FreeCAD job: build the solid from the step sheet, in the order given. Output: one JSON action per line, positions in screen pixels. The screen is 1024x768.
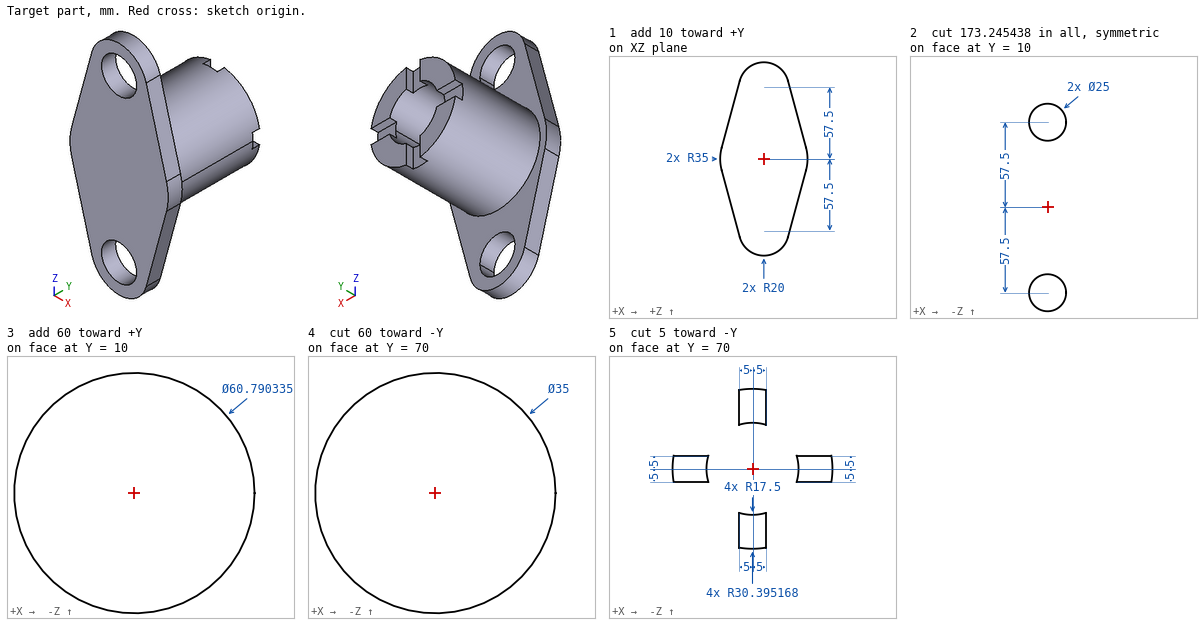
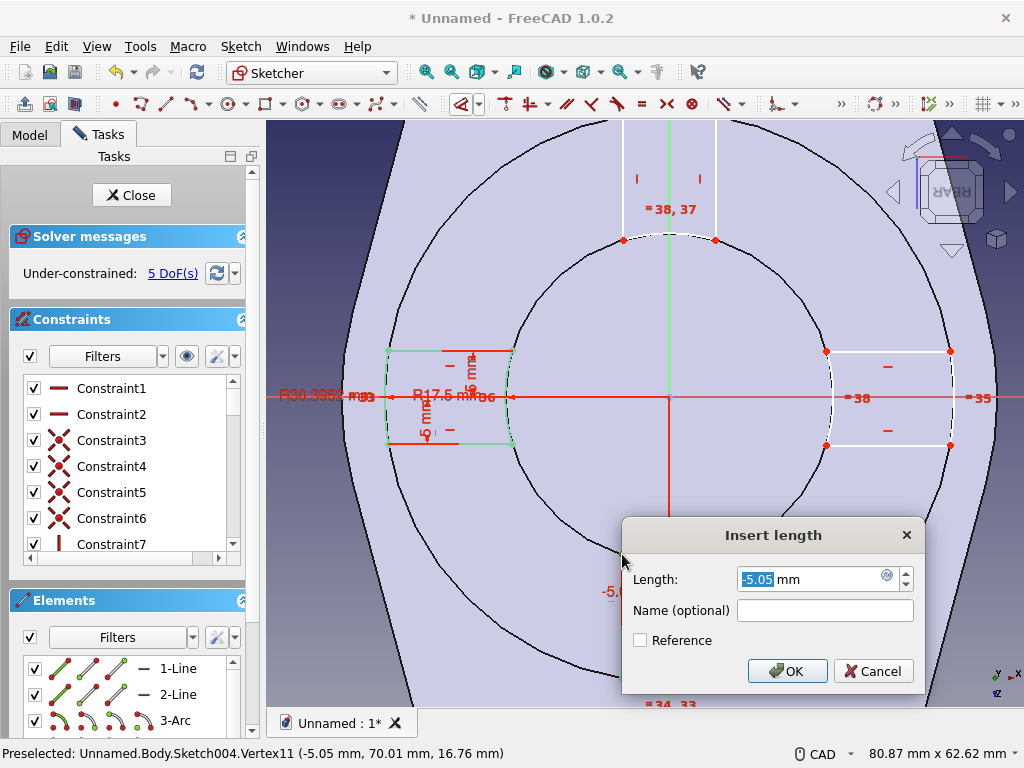
{"action": "type", "text": "-5"}
{"action": "key", "text": "Return"}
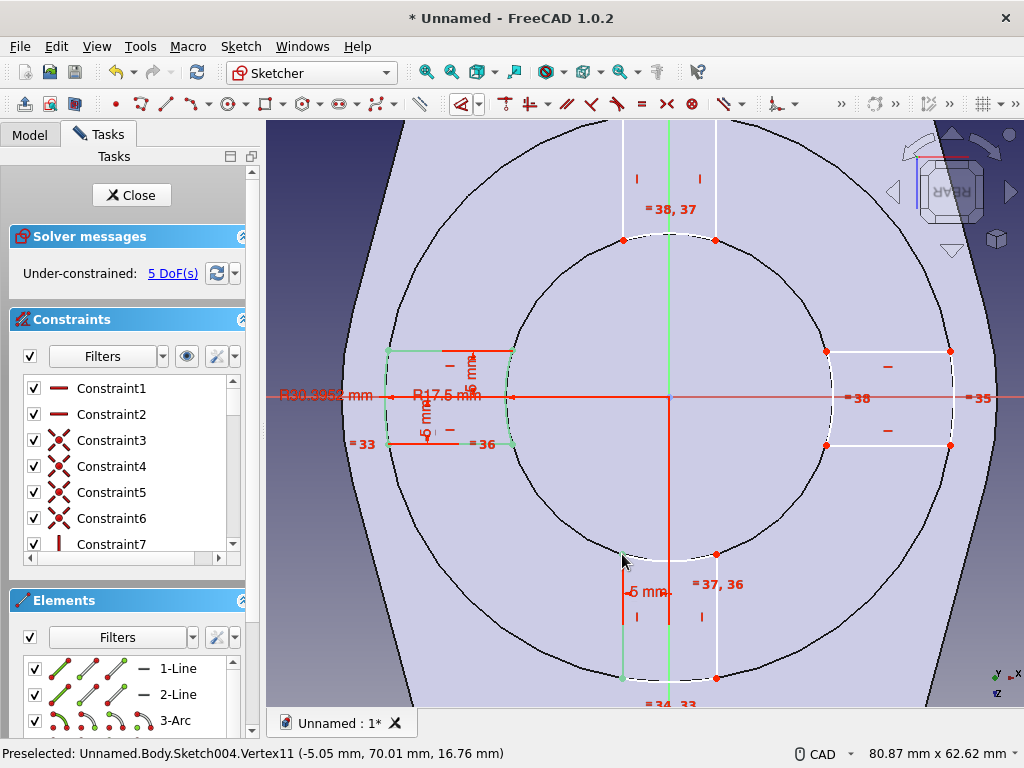
{"action": "left_click", "coordinate": [717, 678]}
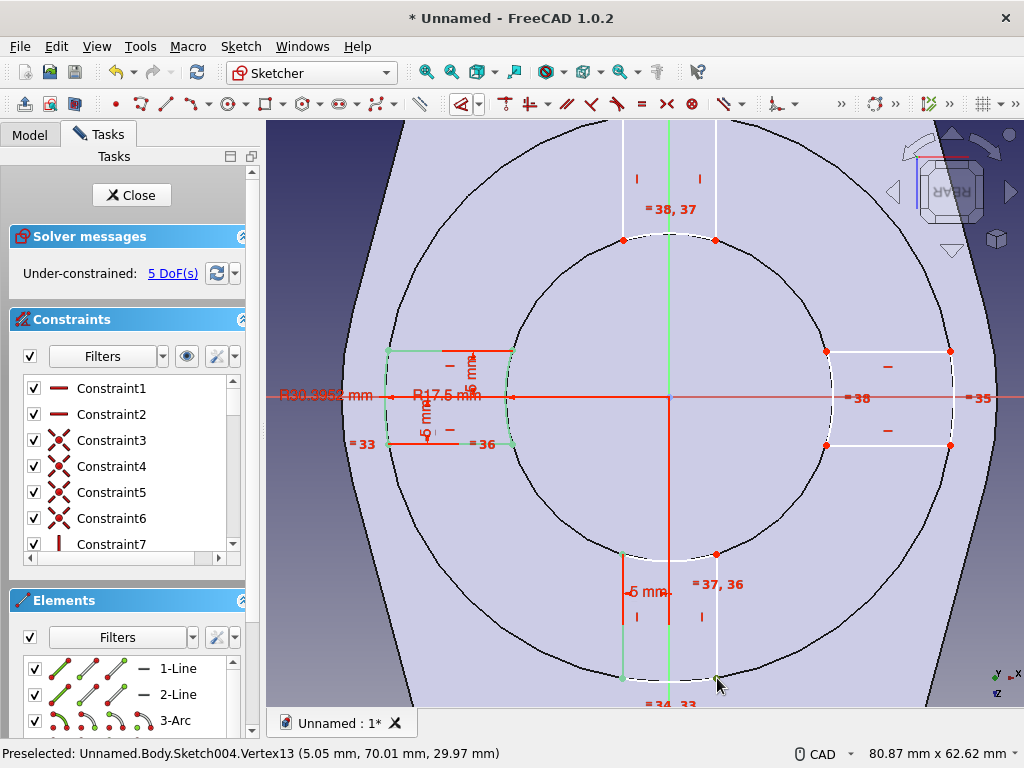
{"action": "left_click", "coordinate": [478, 104]}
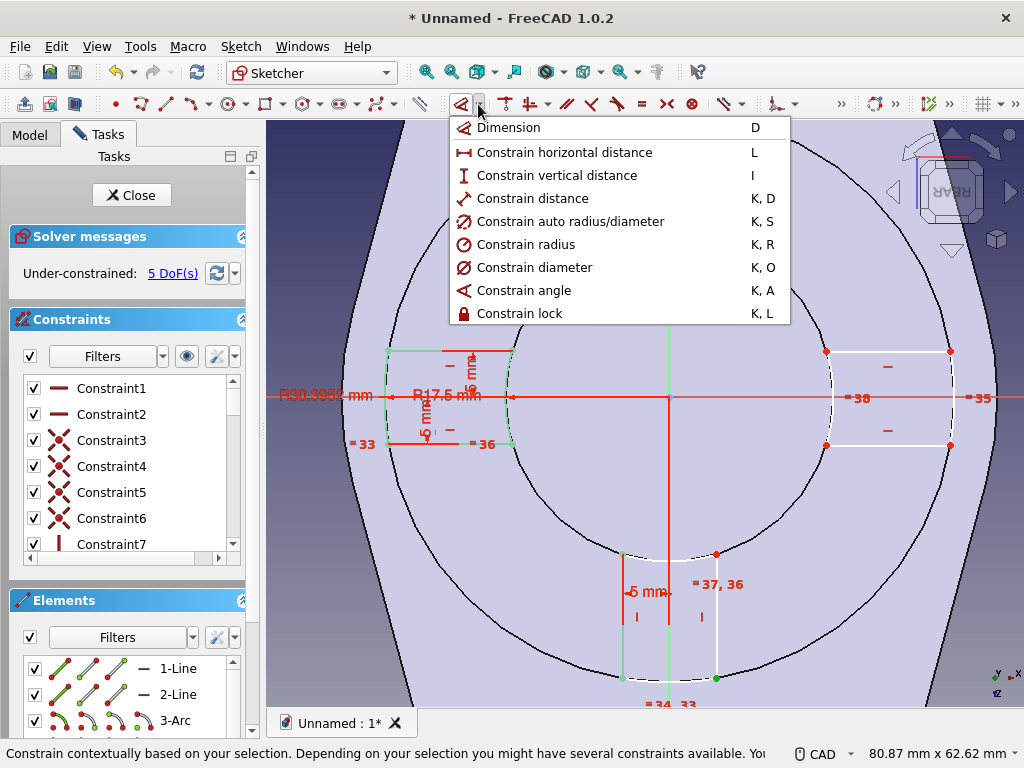
{"action": "left_click", "coordinate": [620, 152]}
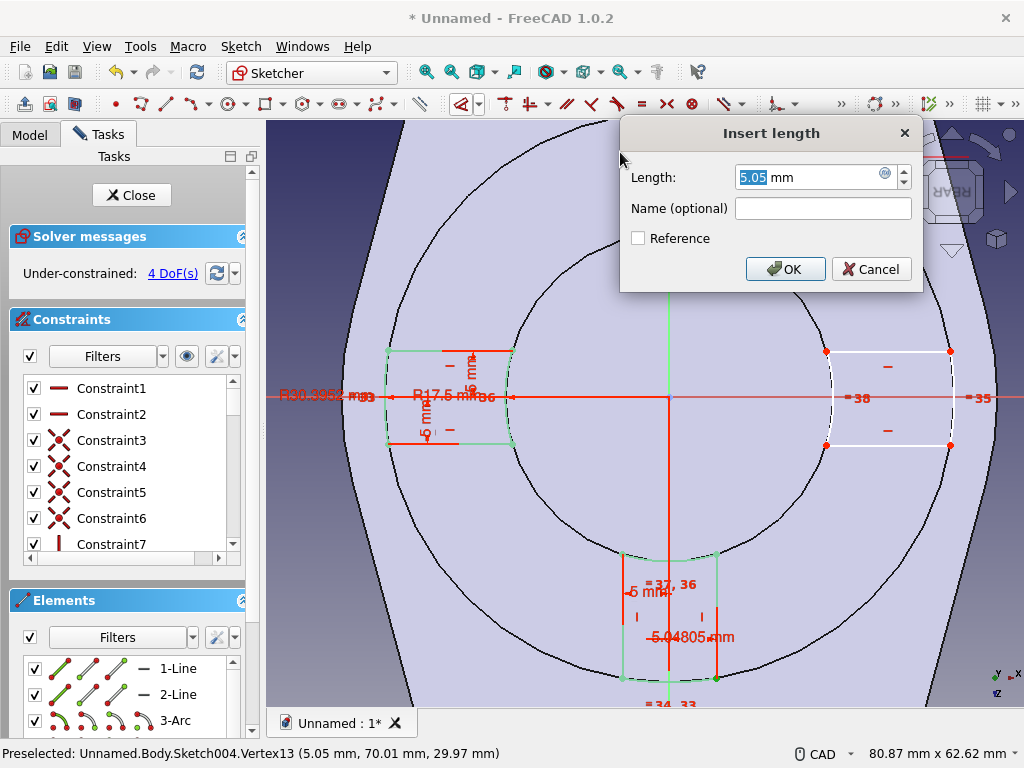
{"action": "type", "text": "5"}
{"action": "key", "text": "Return"}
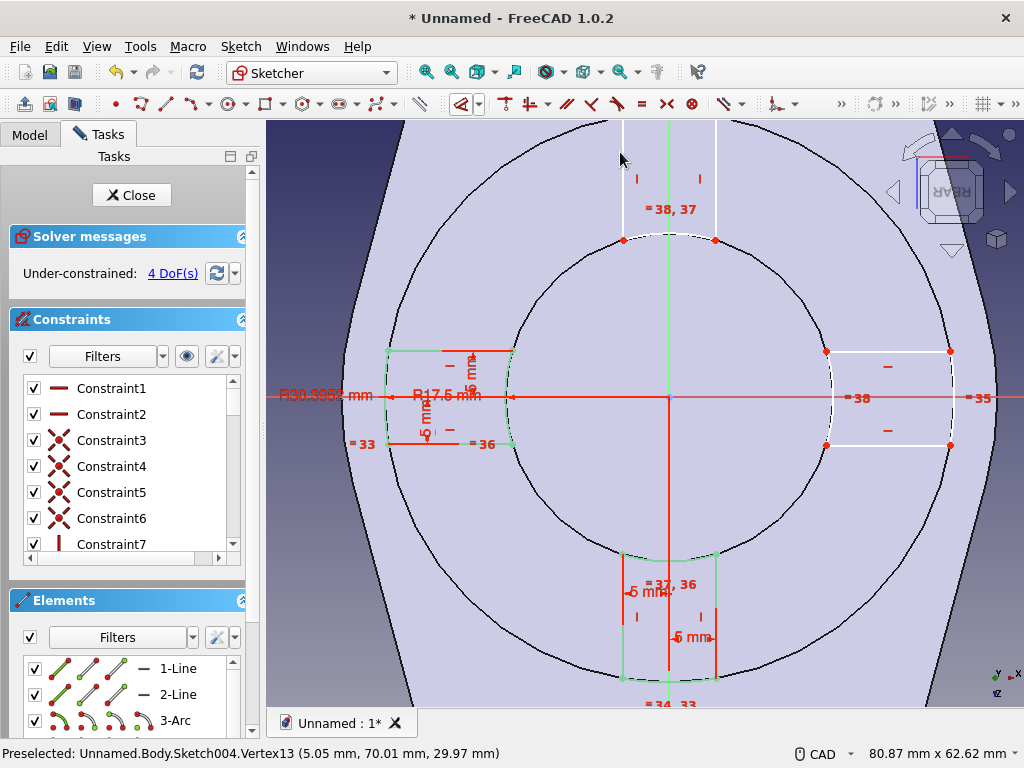
{"action": "scroll", "coordinate": [388, 446], "scroll_direction": "down", "scroll_amount": 2}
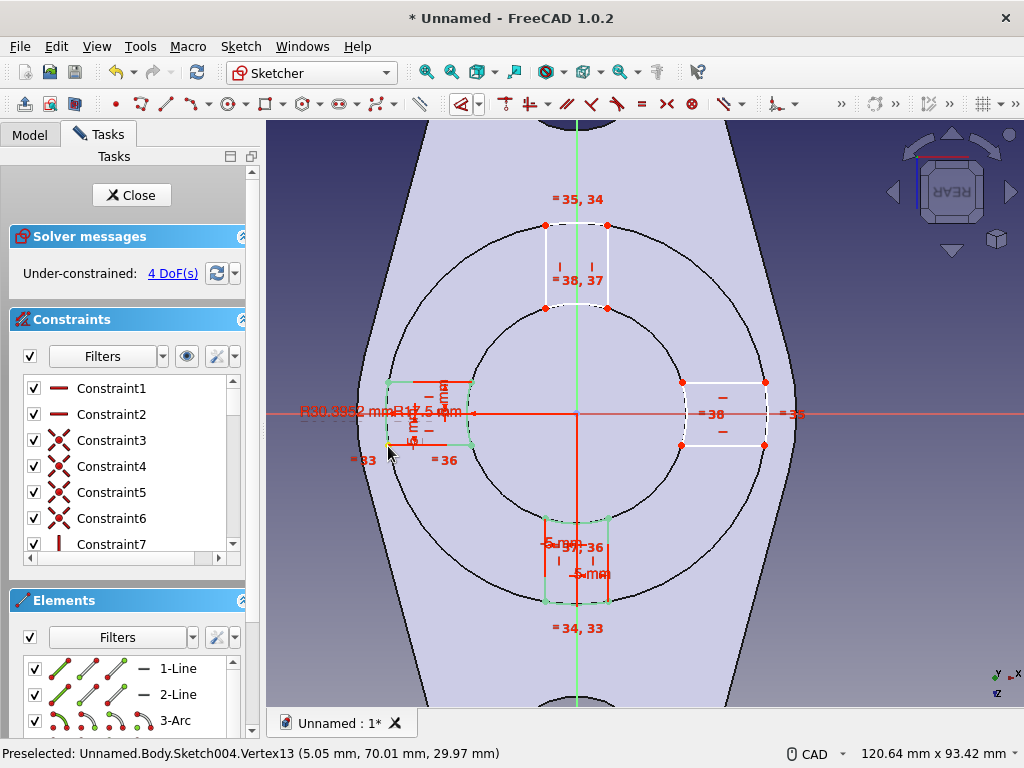
{"action": "scroll", "coordinate": [546, 225], "scroll_direction": "up", "scroll_amount": 2}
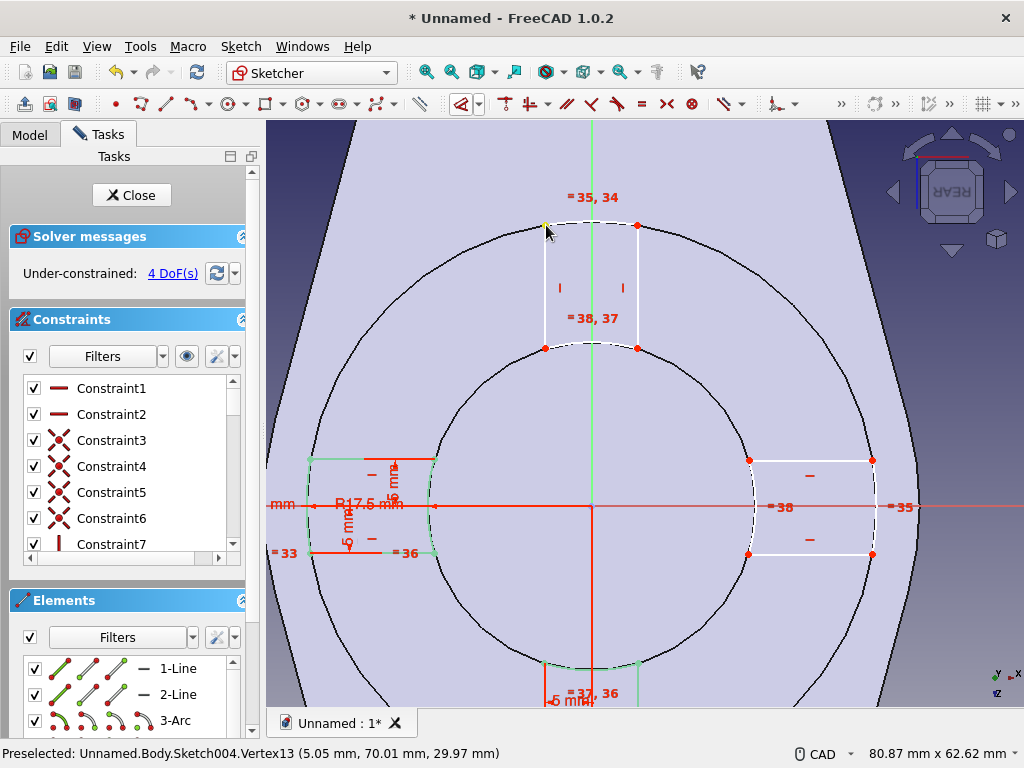
{"action": "left_click", "coordinate": [545, 225]}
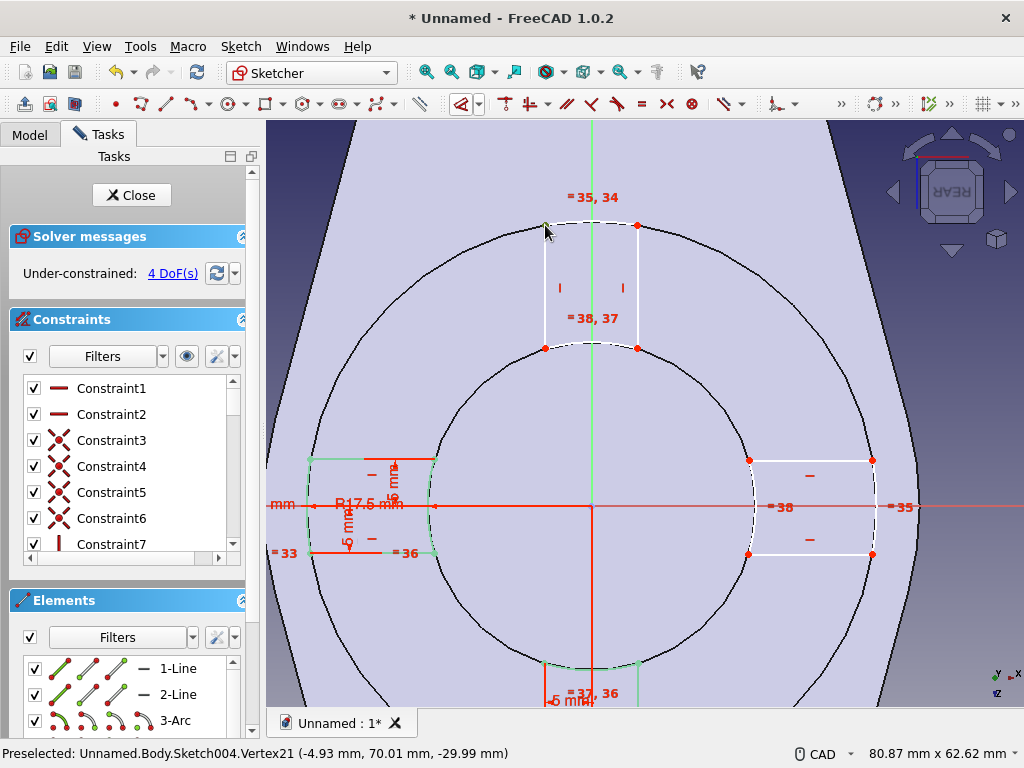
{"action": "key", "text": "l"}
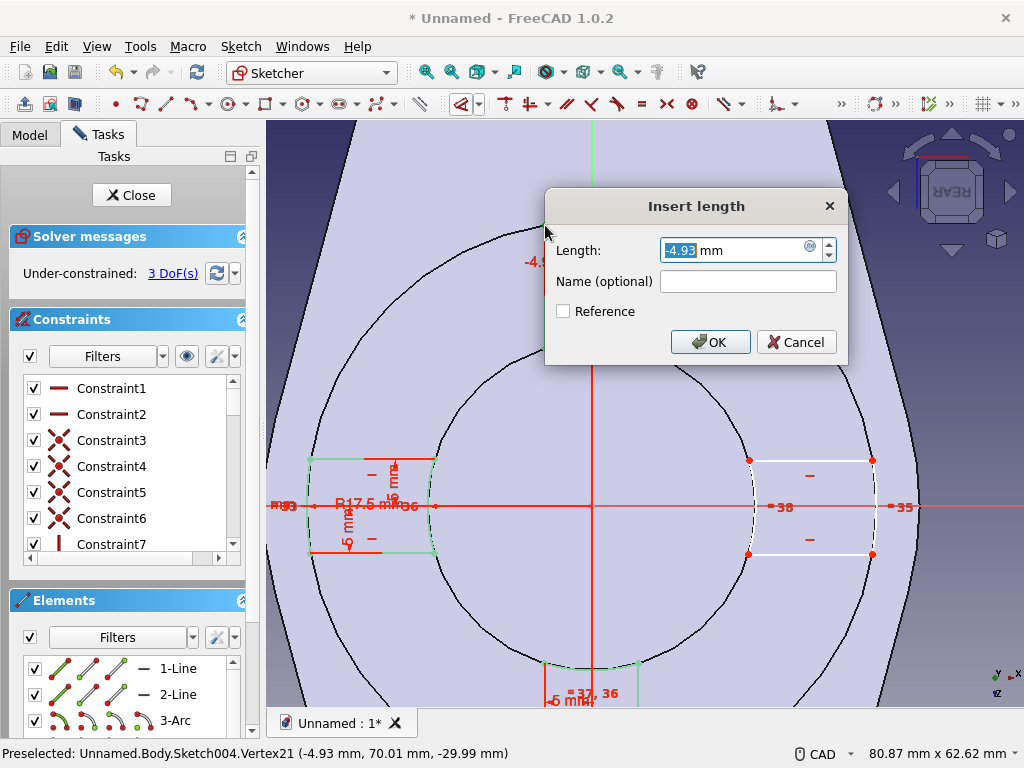
{"action": "type", "text": "-5"}
{"action": "key", "text": "Return"}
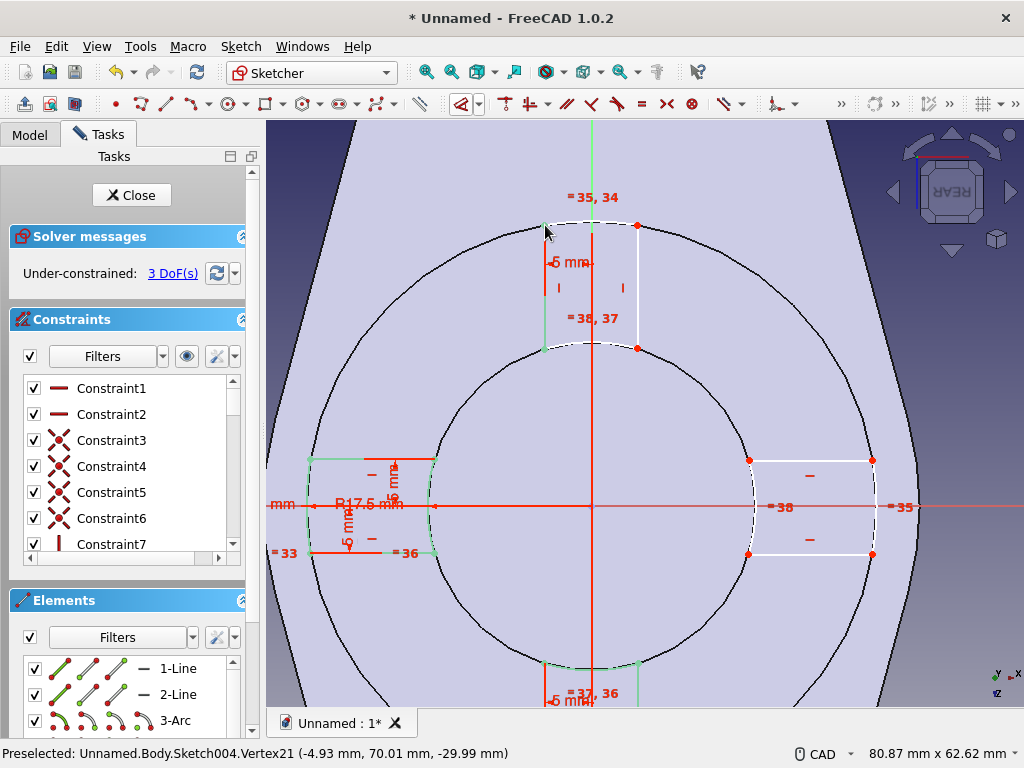
{"action": "left_click", "coordinate": [638, 349]}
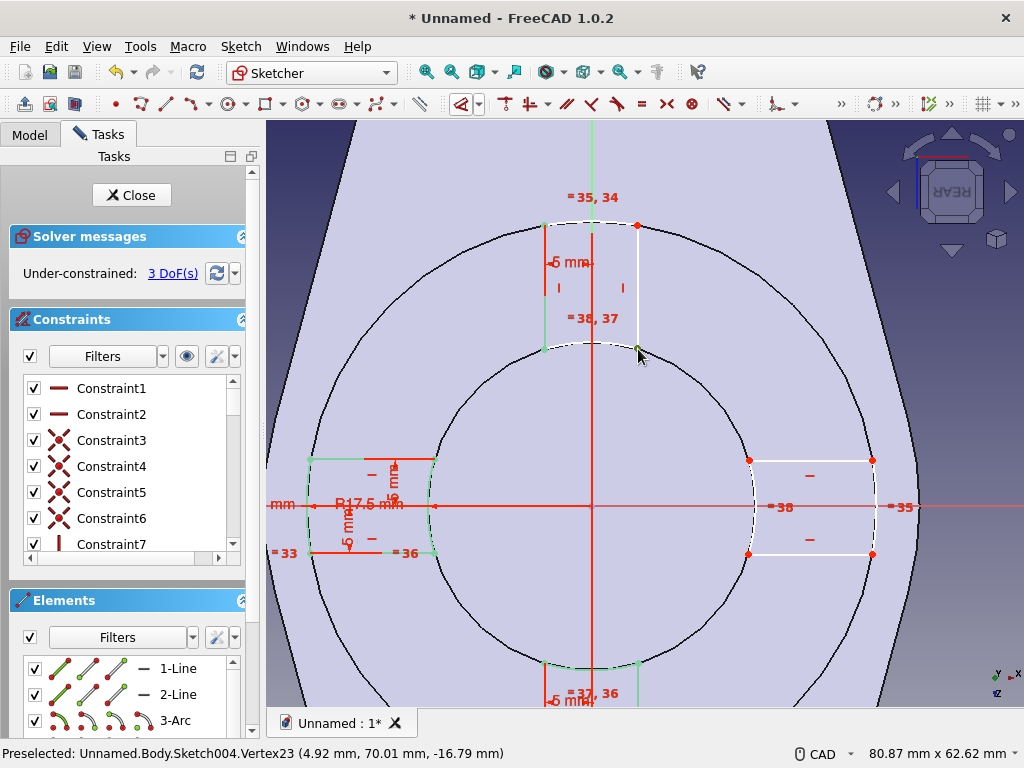
{"action": "key", "text": "l"}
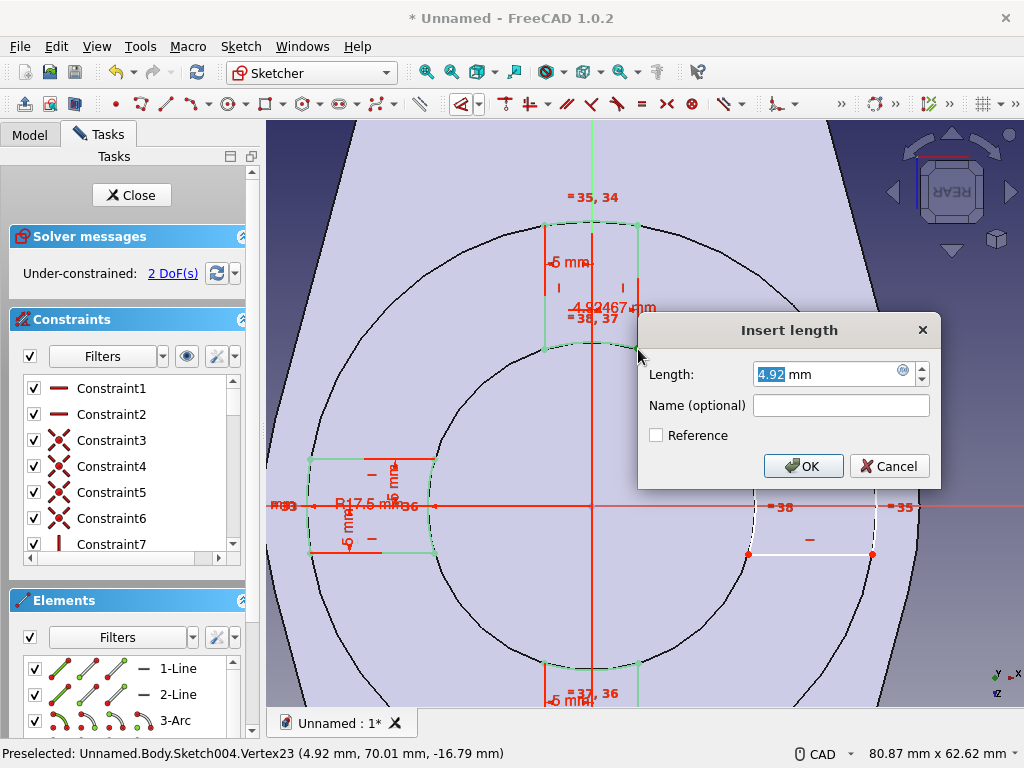
{"action": "type", "text": "5"}
{"action": "key", "text": "Return"}